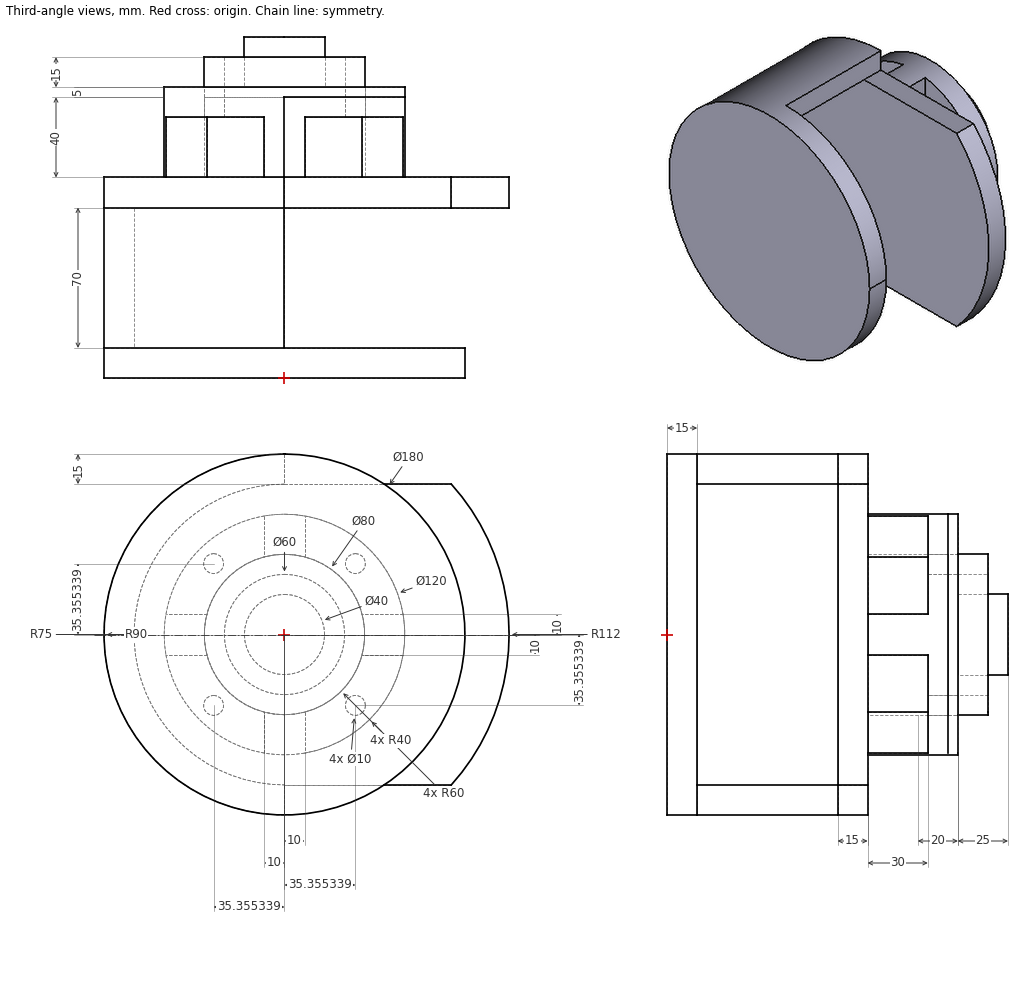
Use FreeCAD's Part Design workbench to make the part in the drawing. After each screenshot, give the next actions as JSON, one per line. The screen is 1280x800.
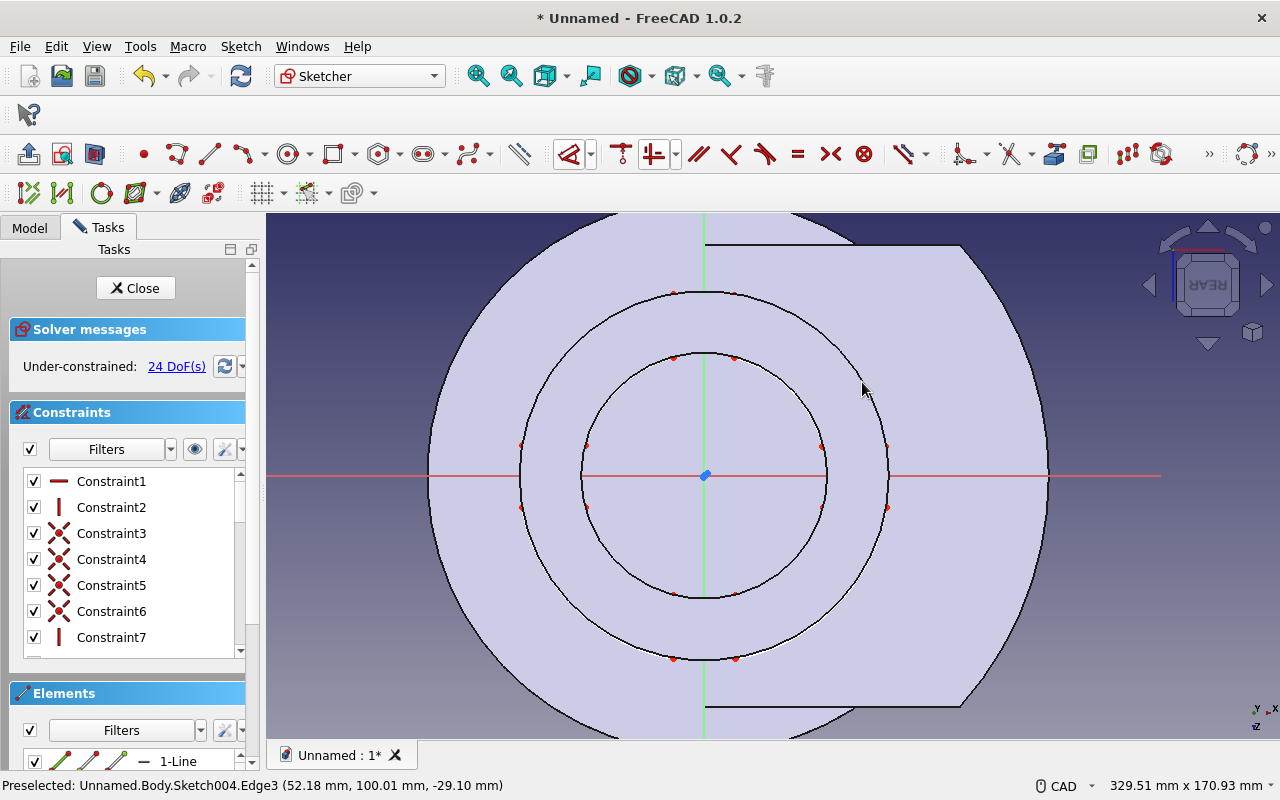
{"action": "left_click", "coordinate": [799, 635]}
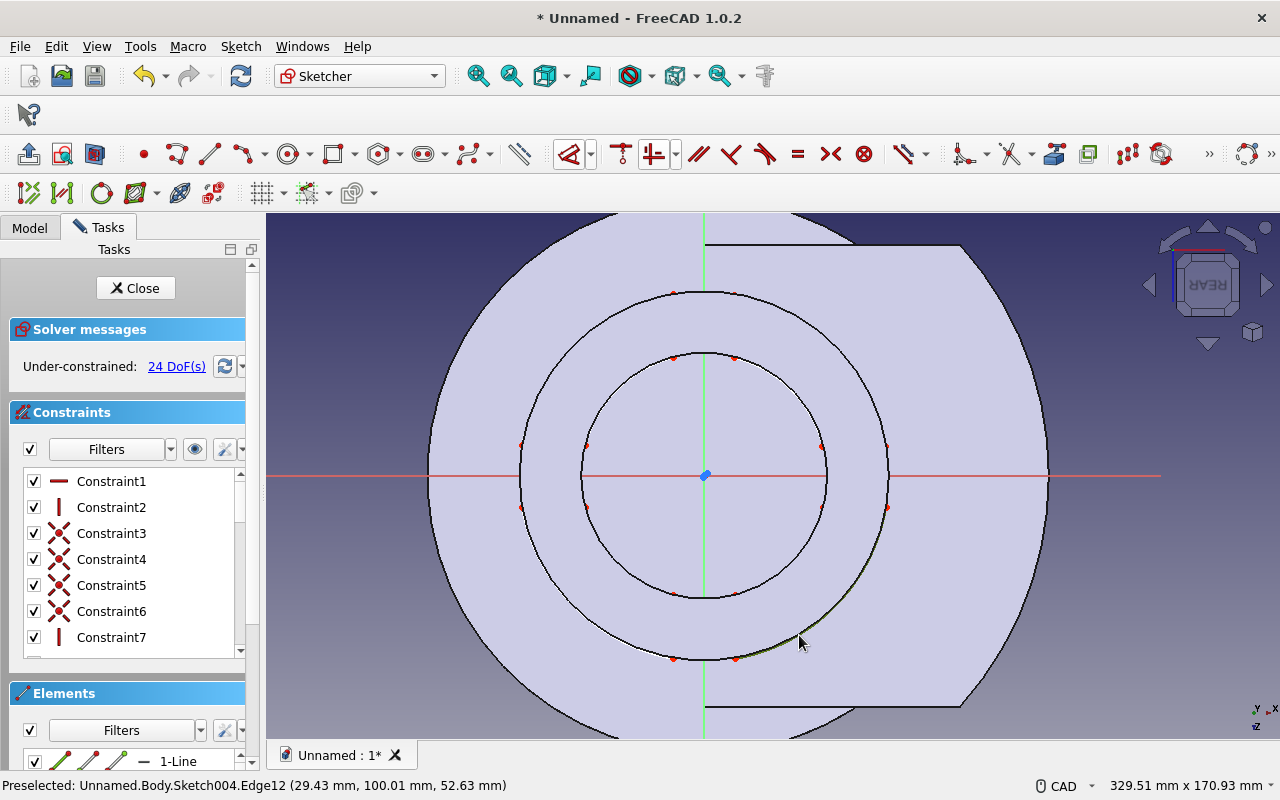
{"action": "left_click", "coordinate": [621, 154]}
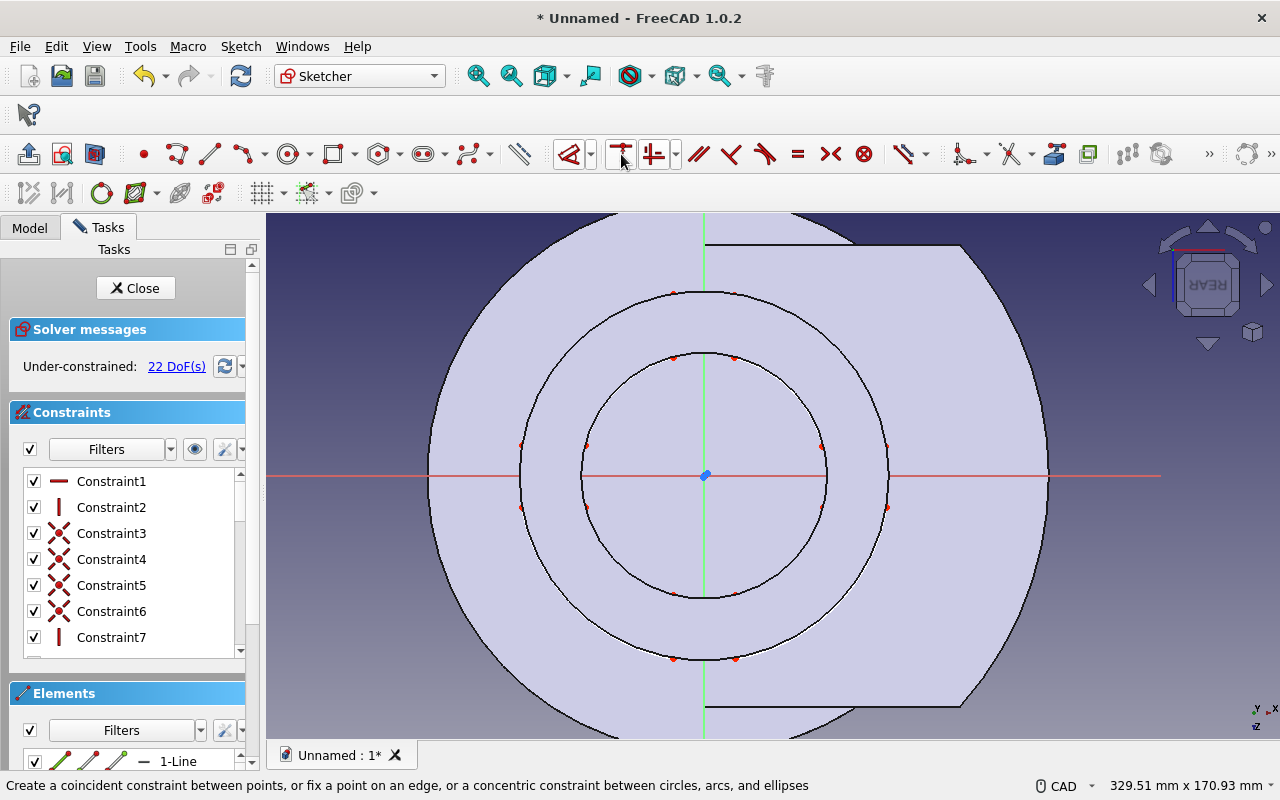
{"action": "left_click", "coordinate": [862, 382]}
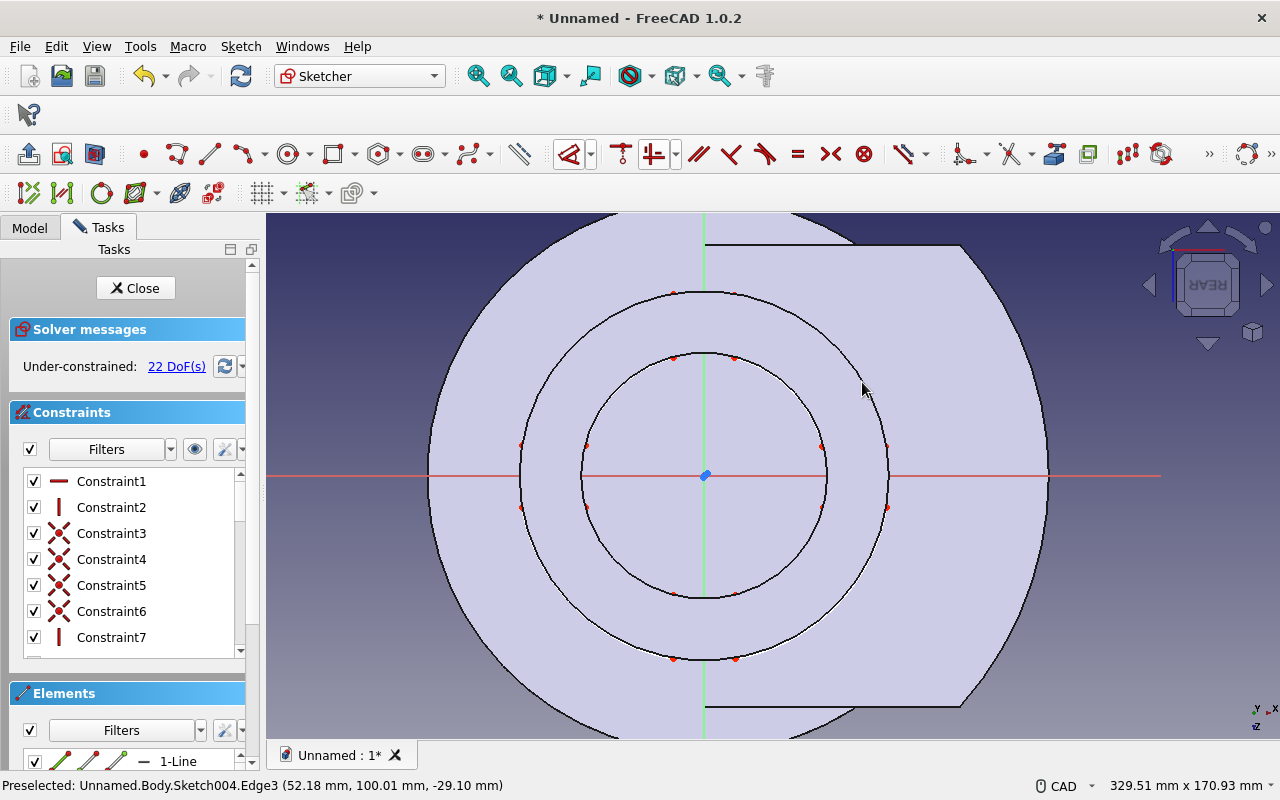
{"action": "left_click", "coordinate": [601, 544]}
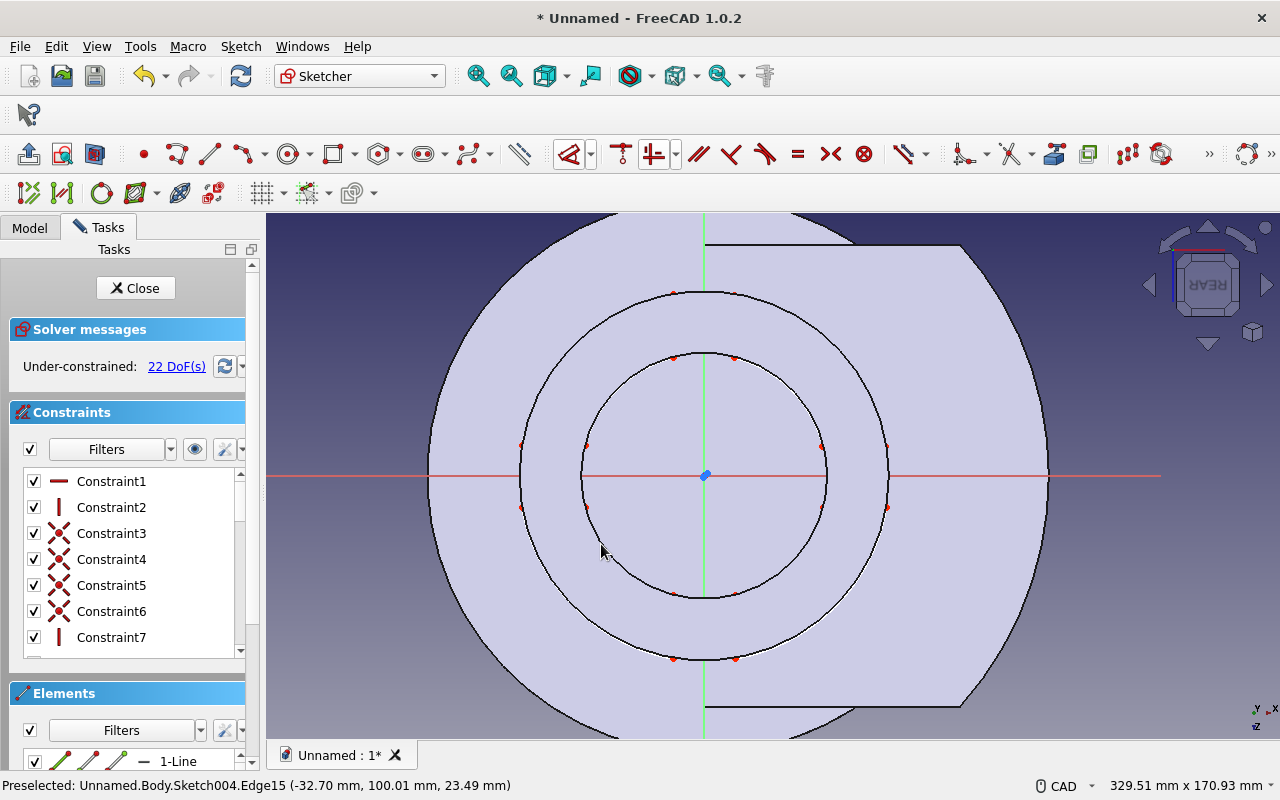
{"action": "key", "text": "c"}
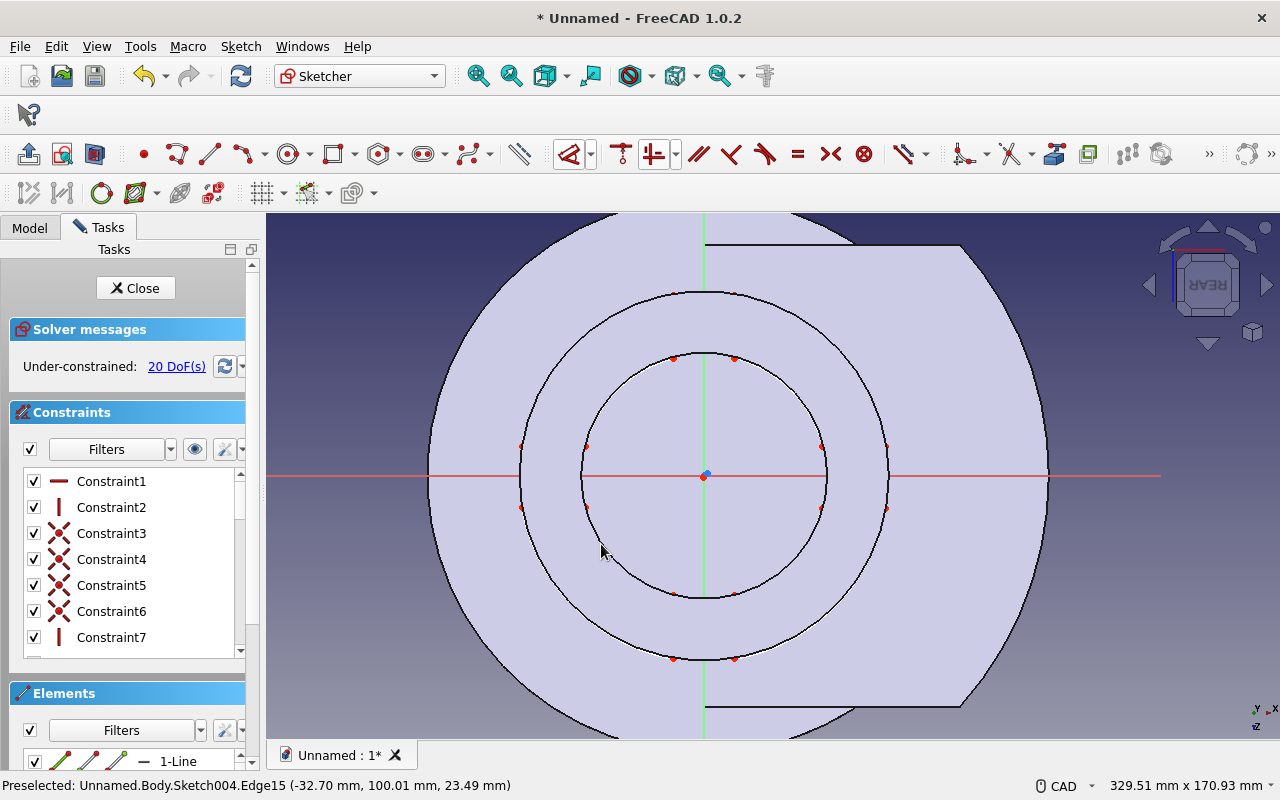
{"action": "left_click", "coordinate": [862, 382]}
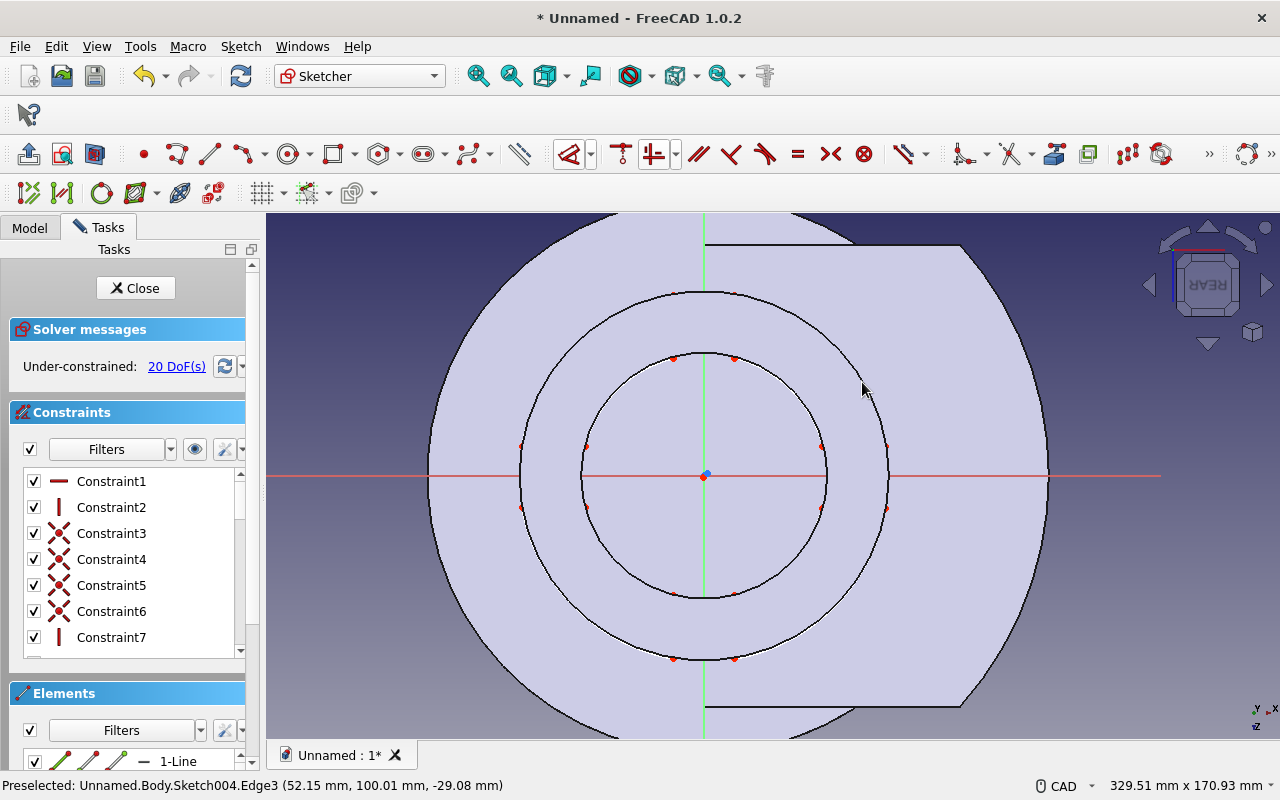
{"action": "left_click", "coordinate": [546, 571]}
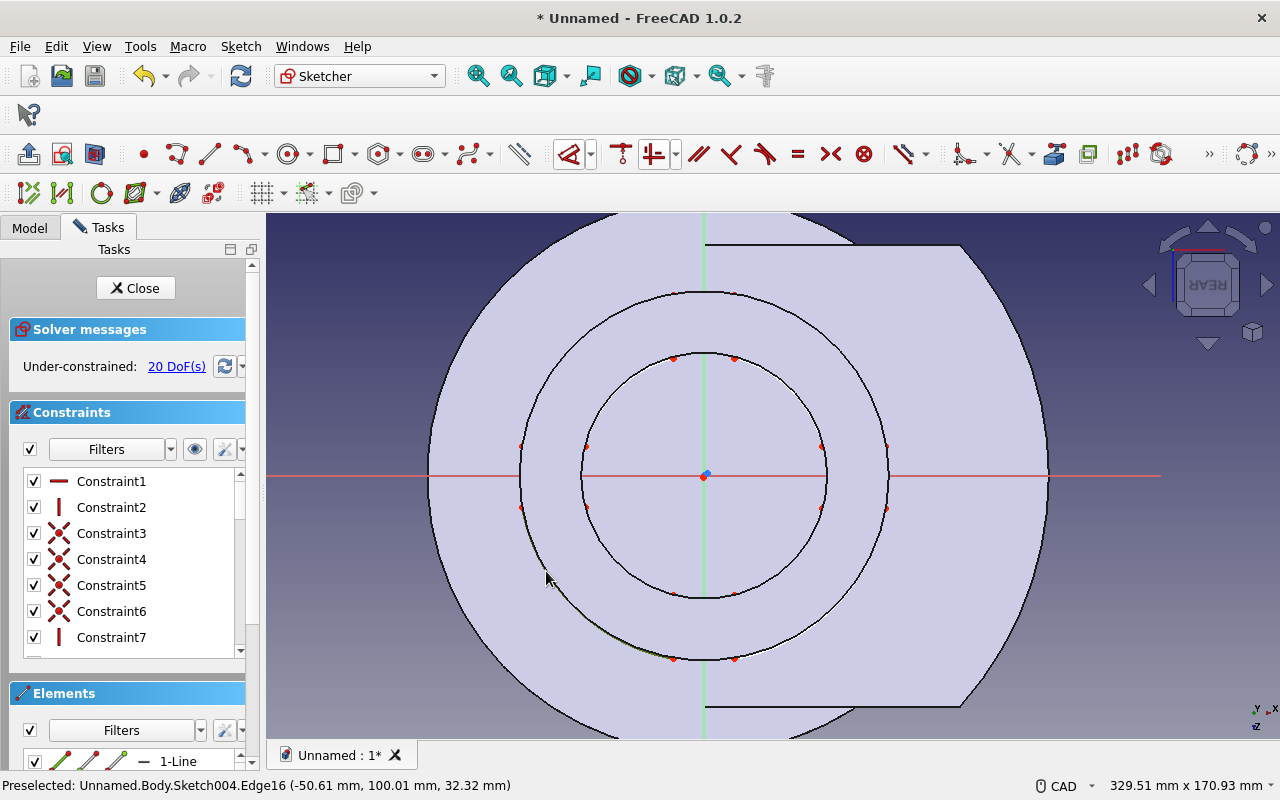
{"action": "left_click", "coordinate": [621, 154]}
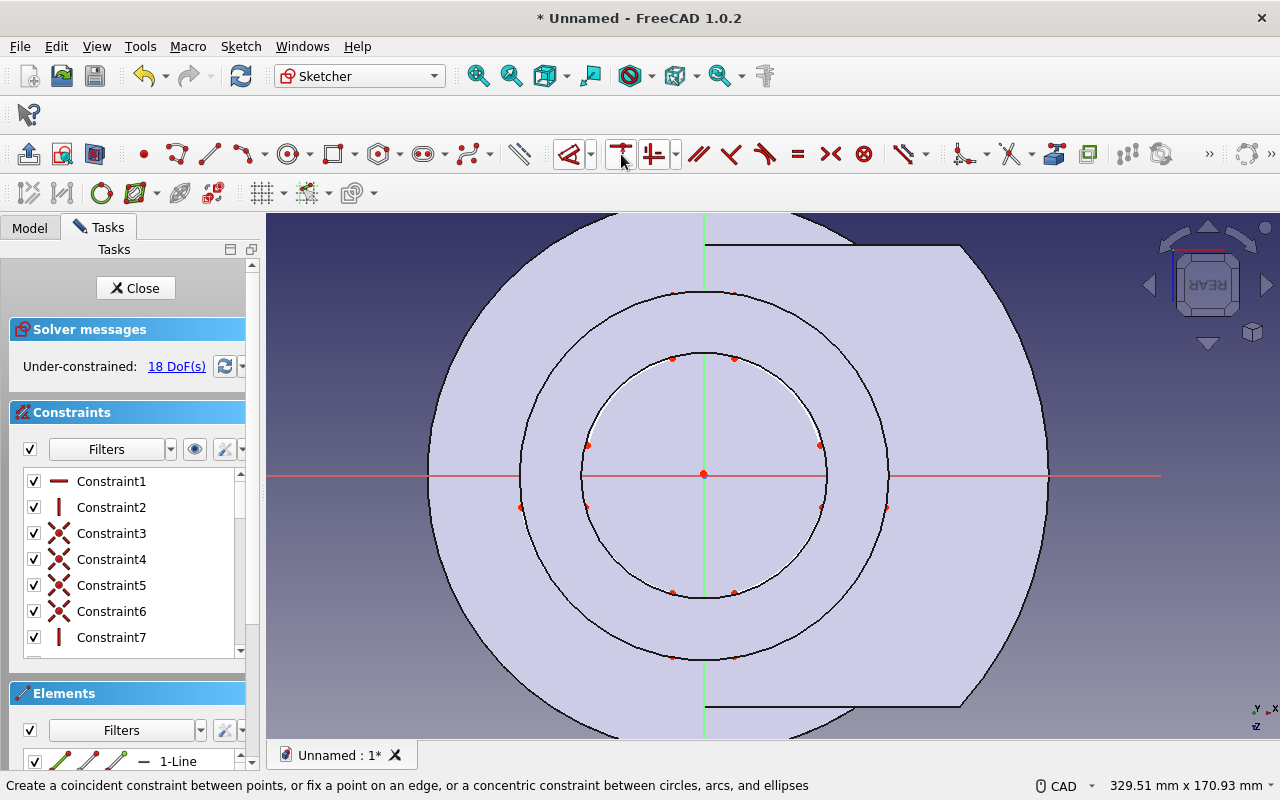
{"action": "left_click_drag", "start_coordinate": [694, 464], "coordinate": [714, 486]}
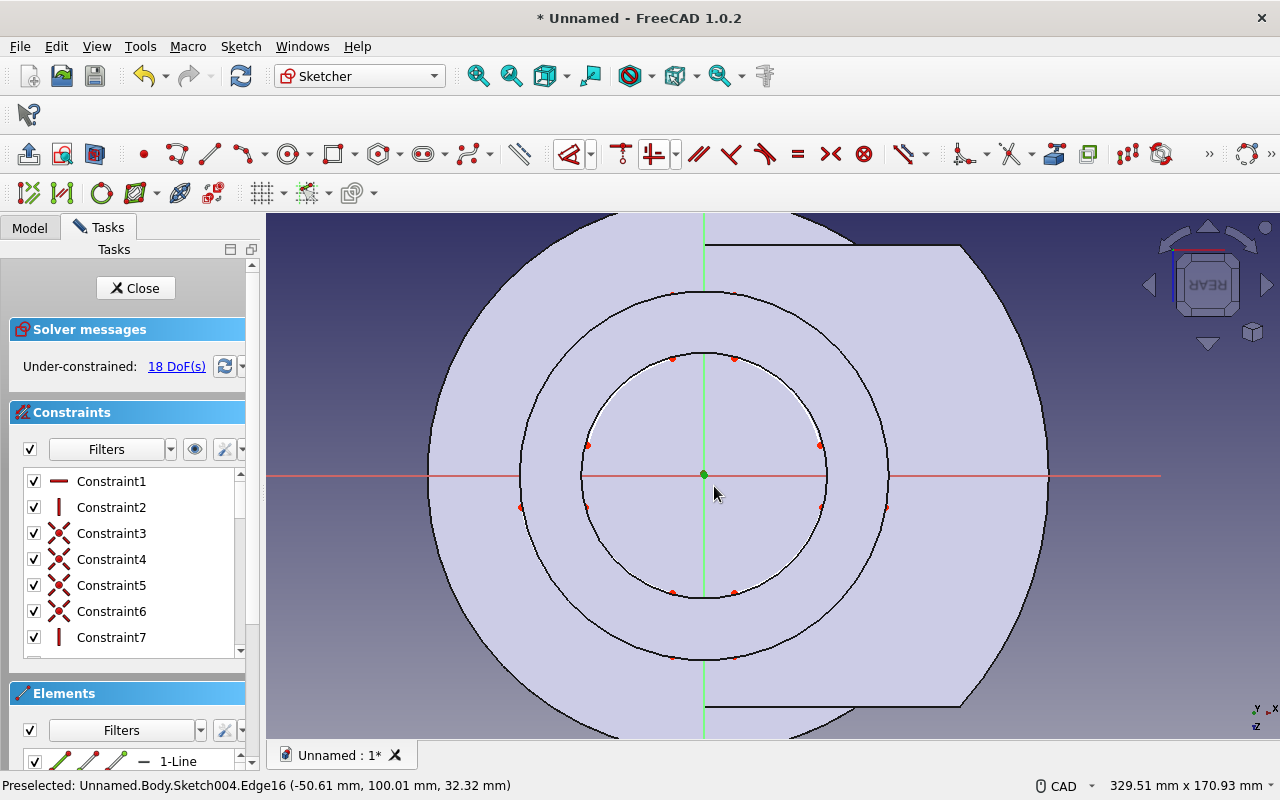
{"action": "left_click", "coordinate": [621, 154]}